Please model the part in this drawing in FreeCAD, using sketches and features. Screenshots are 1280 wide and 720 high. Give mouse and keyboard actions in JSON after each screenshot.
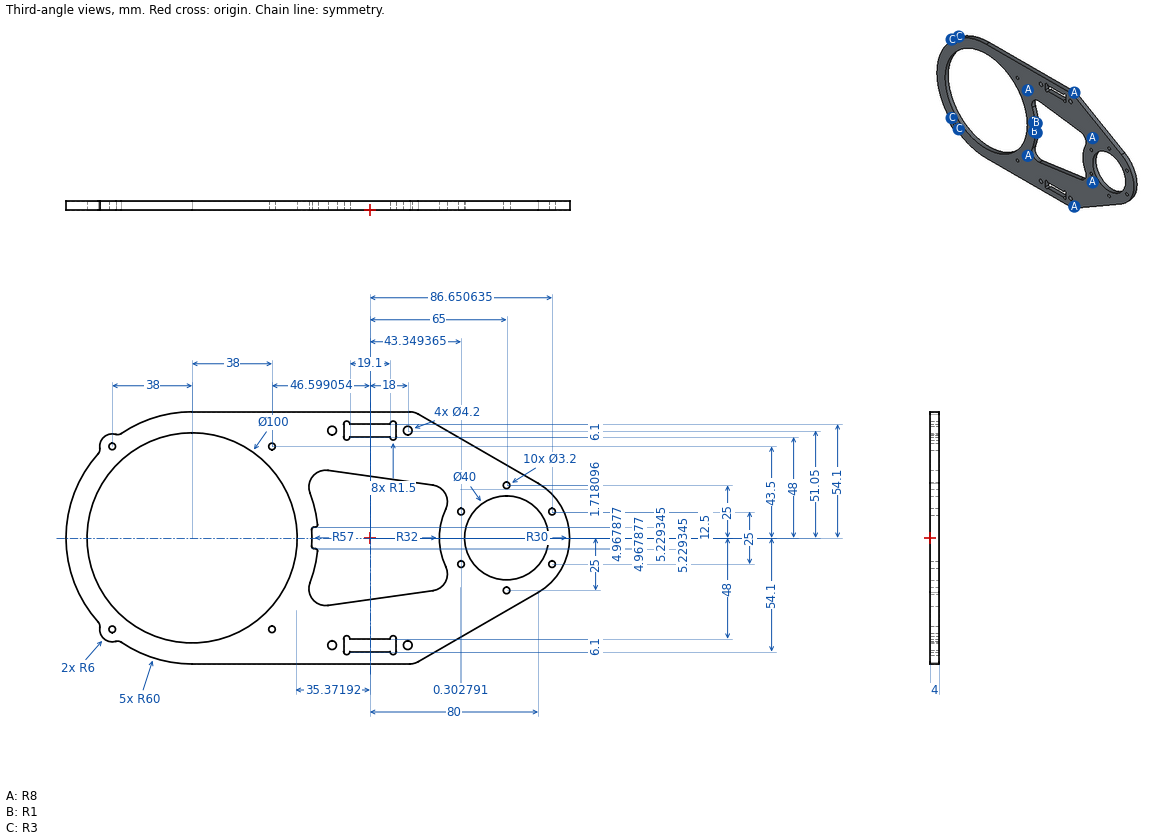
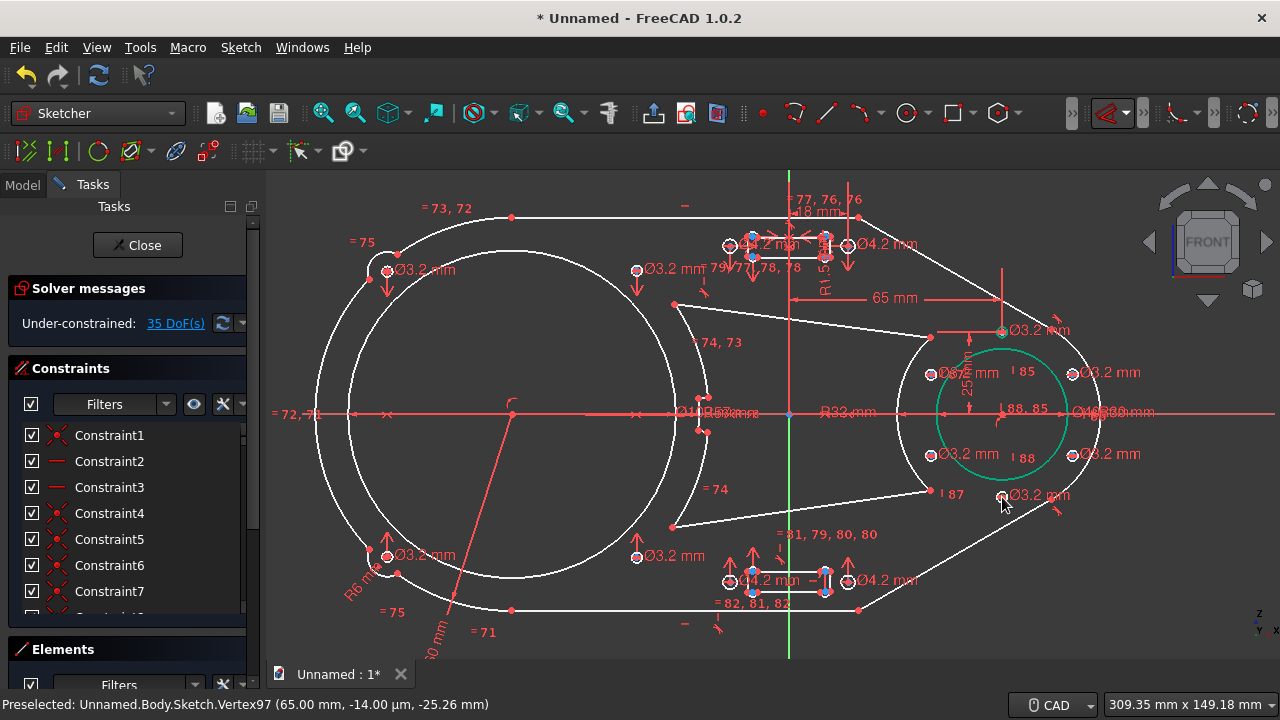
{"action": "left_click", "coordinate": [1128, 114]}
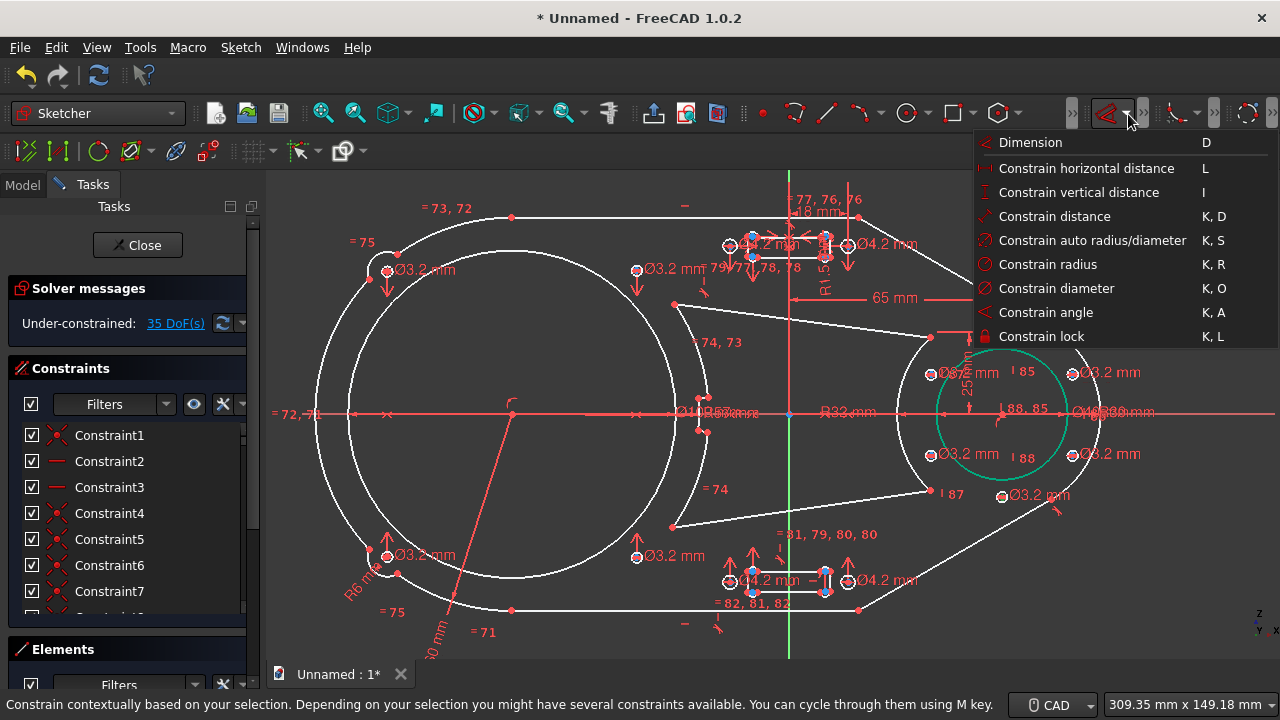
{"action": "left_click", "coordinate": [1126, 192]}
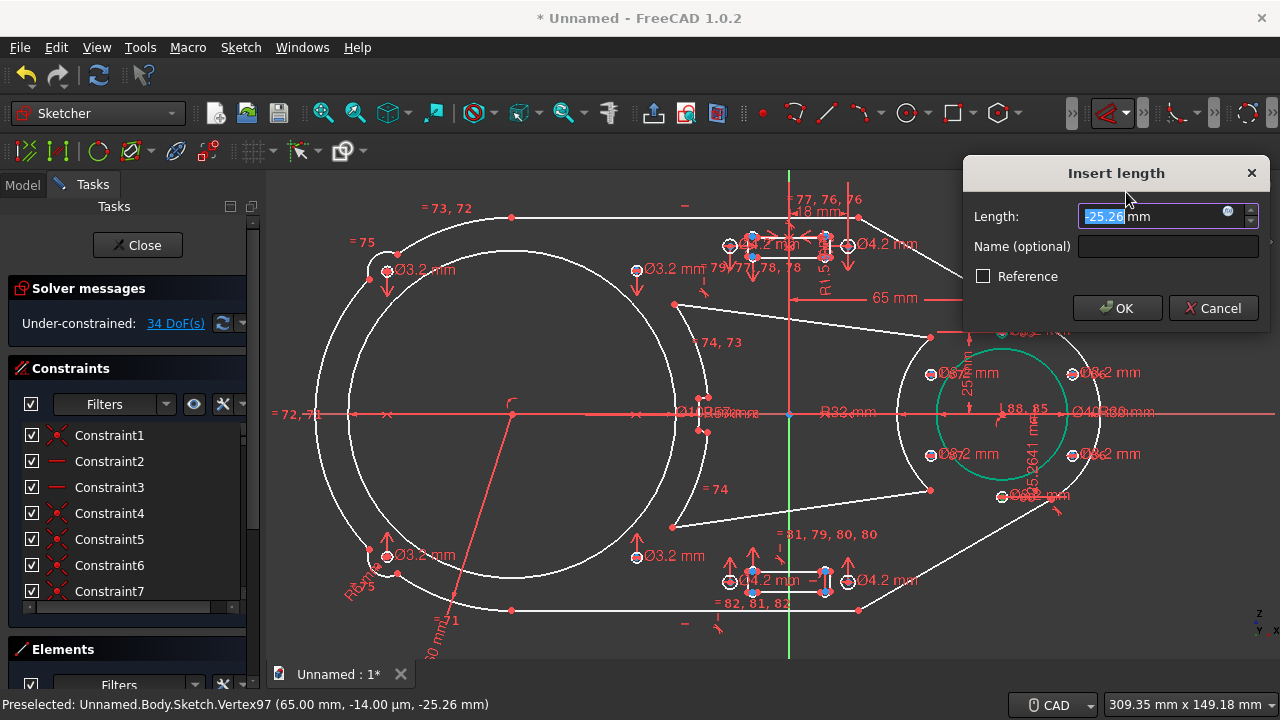
{"action": "type", "text": "-25"}
{"action": "key", "text": "Return"}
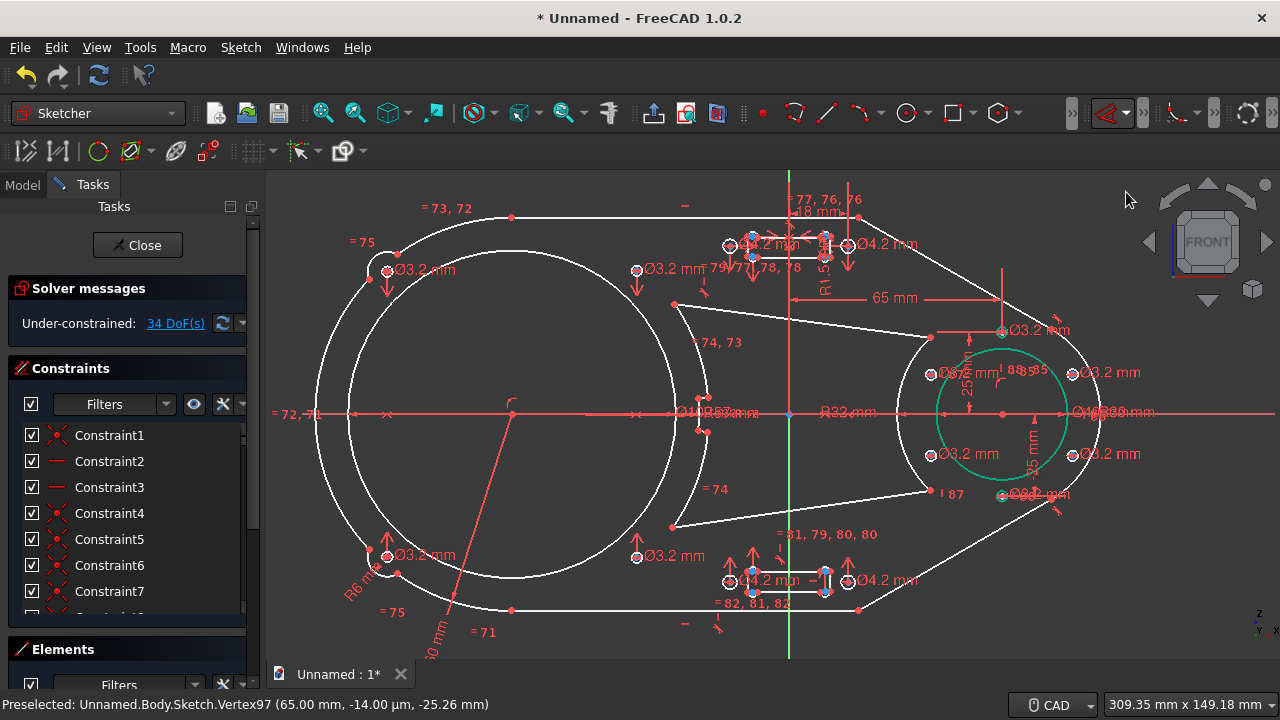
{"action": "scroll", "coordinate": [830, 247], "scroll_direction": "up", "scroll_amount": 4}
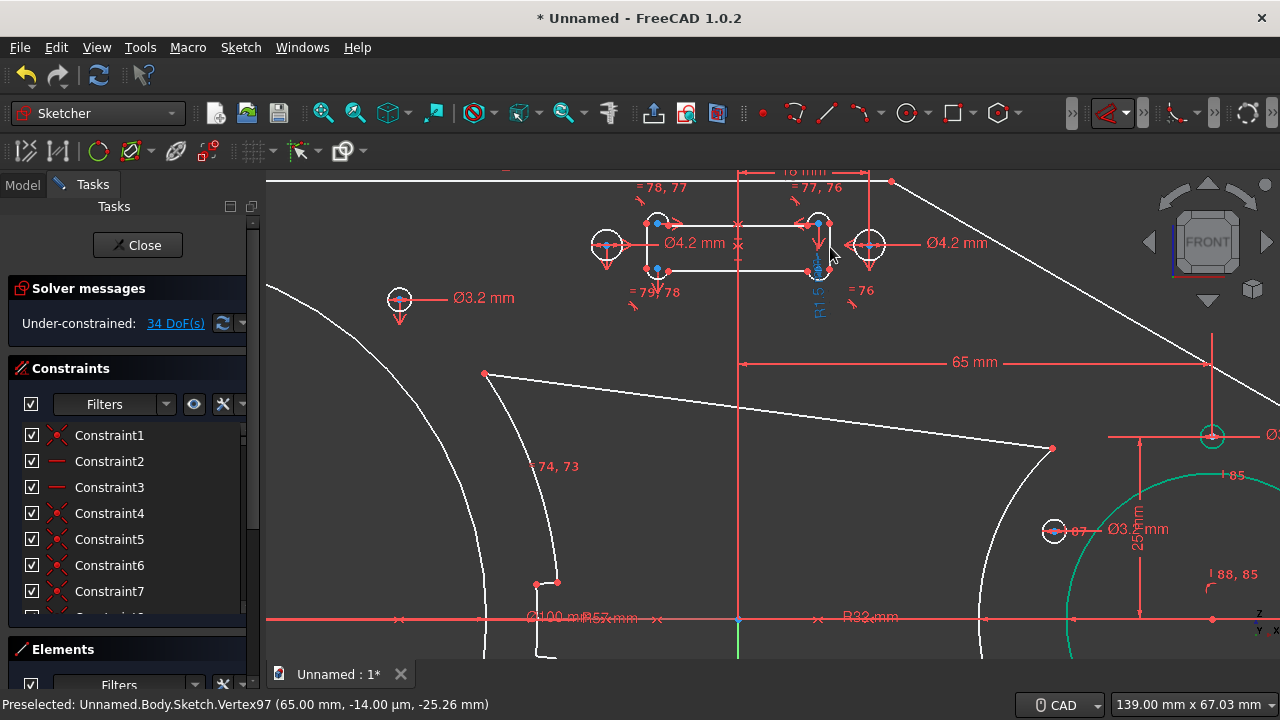
{"action": "left_click", "coordinate": [830, 247]}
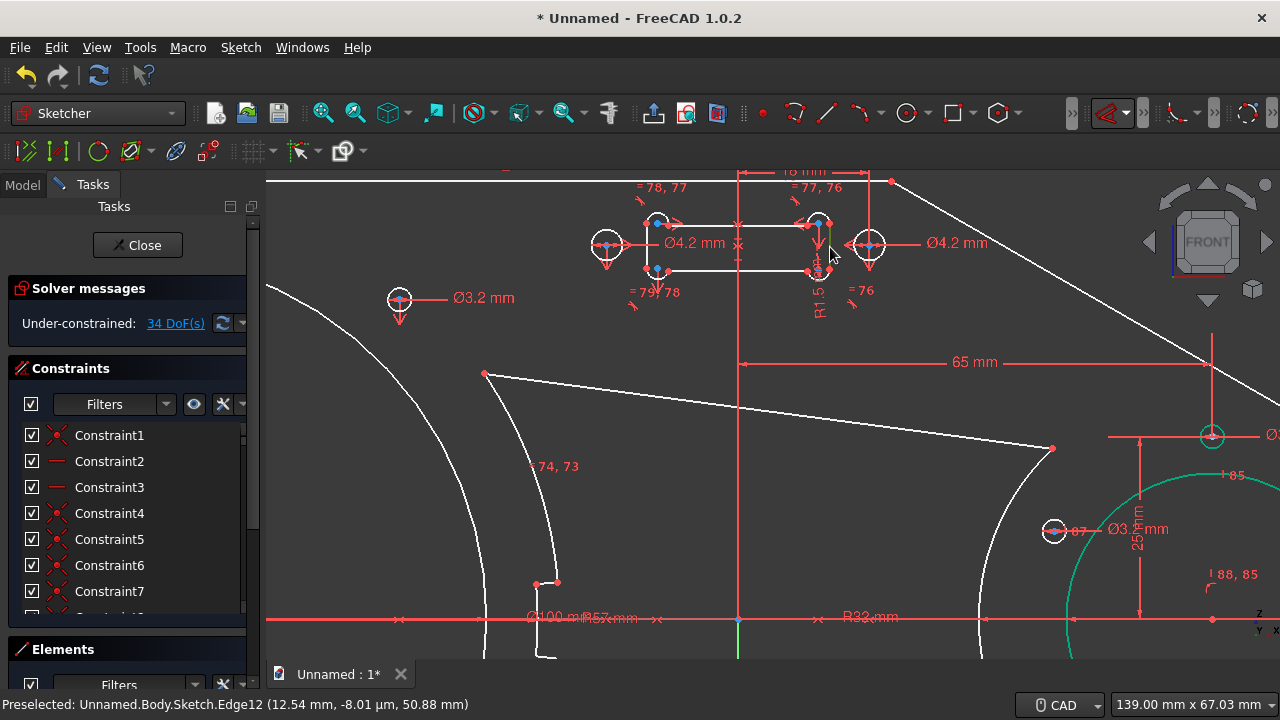
{"action": "key", "text": "i"}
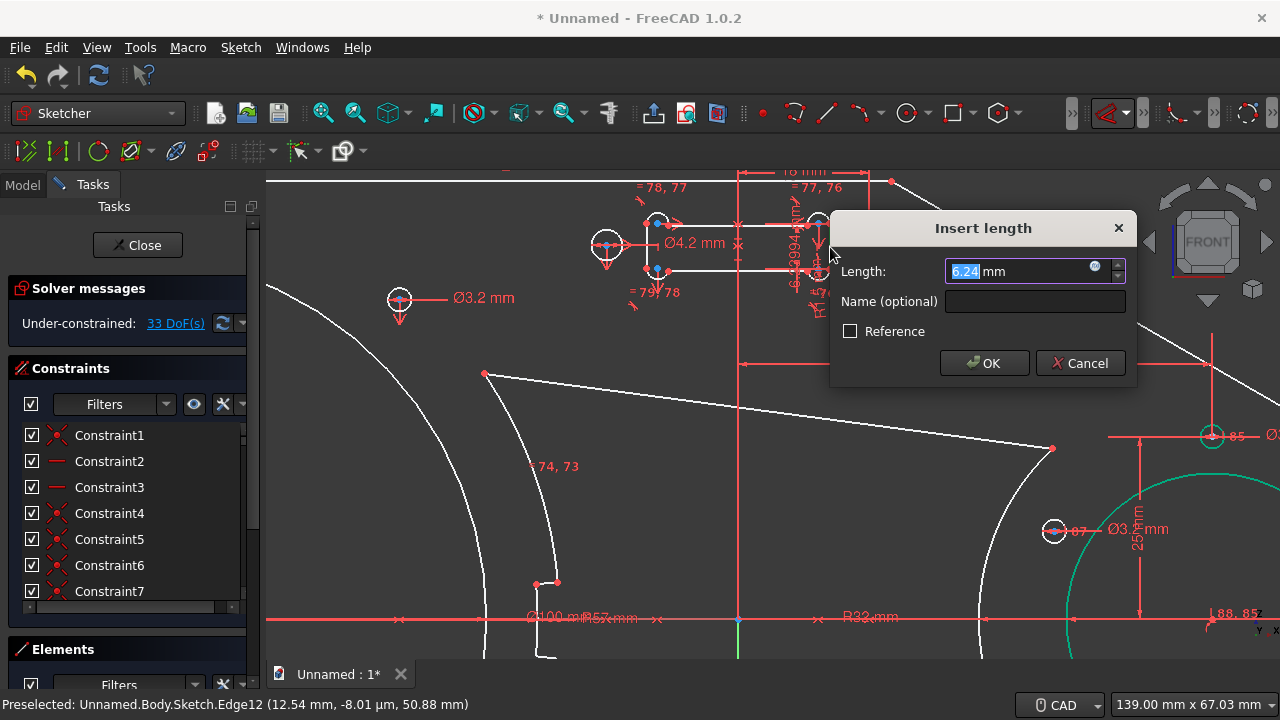
{"action": "type", "text": "6.1"}
{"action": "key", "text": "Return"}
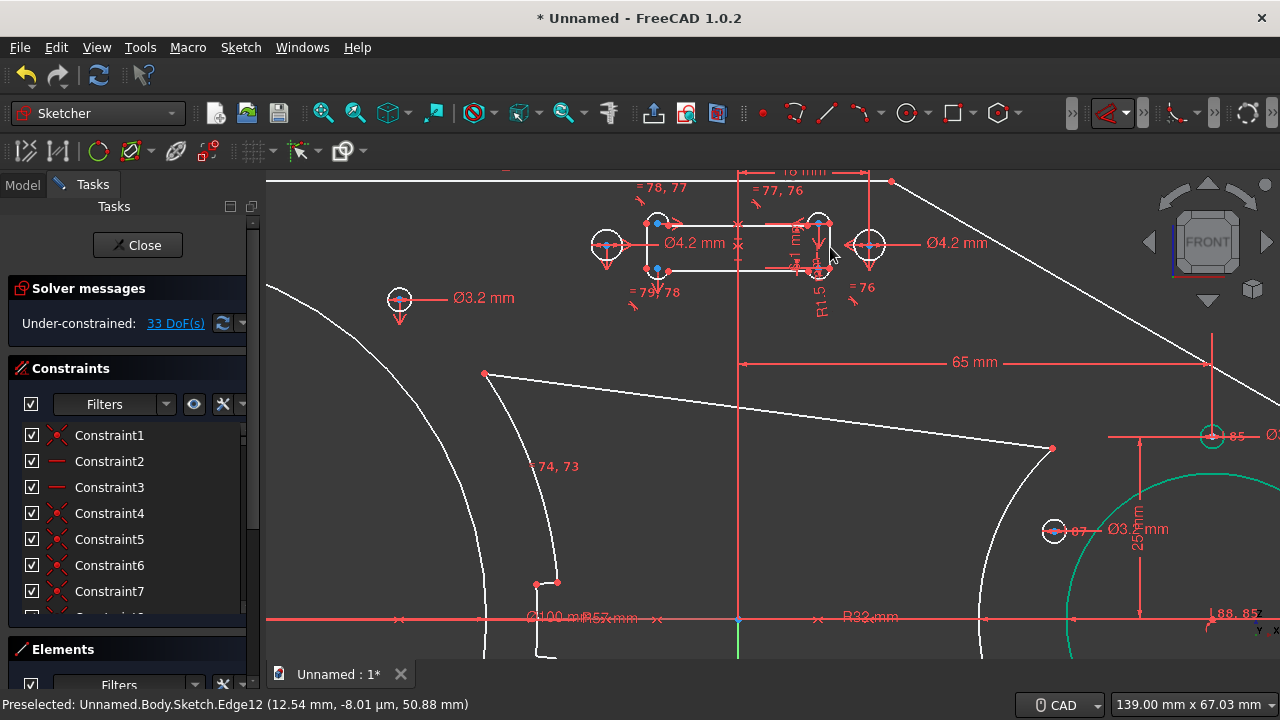
{"action": "left_click", "coordinate": [647, 237]}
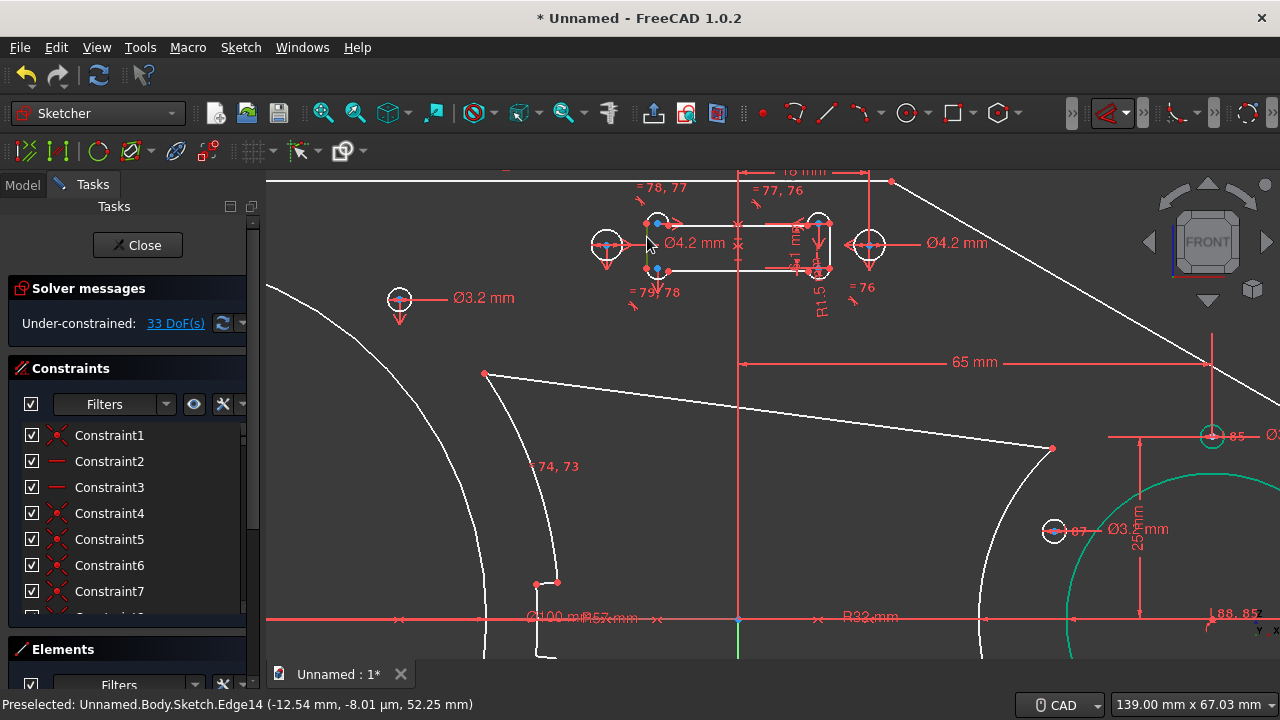
{"action": "left_click", "coordinate": [1128, 114]}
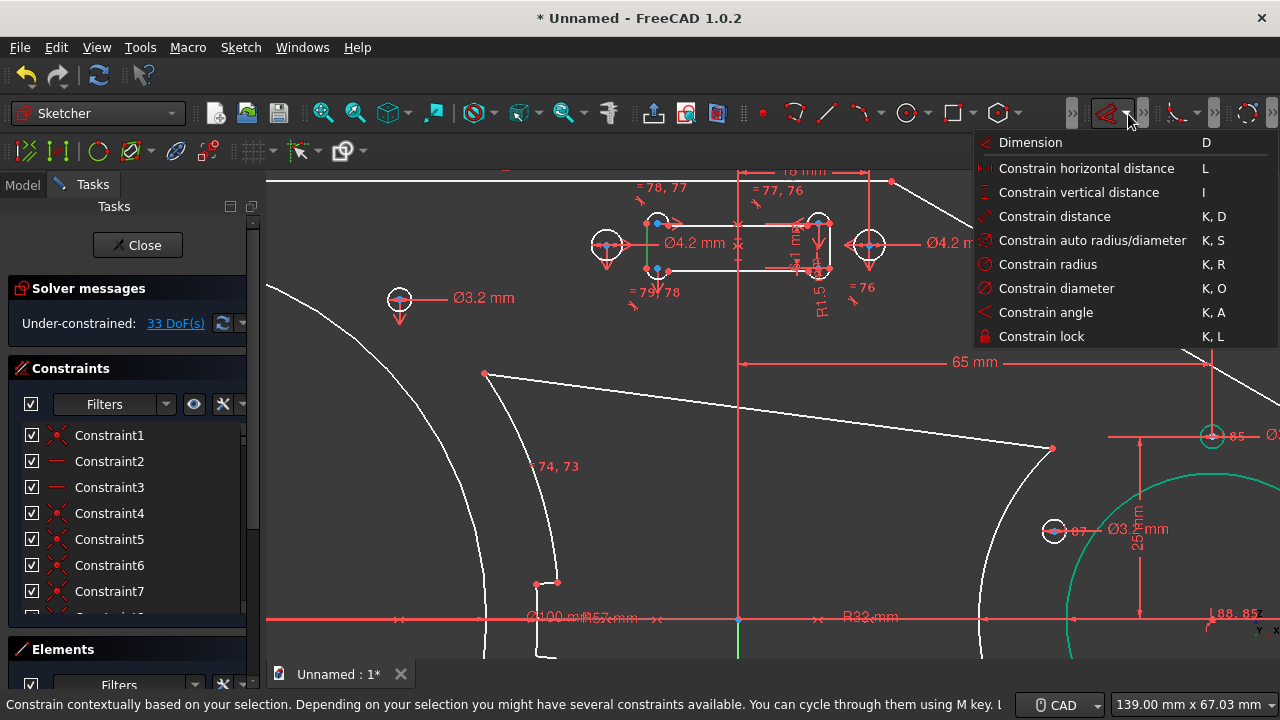
{"action": "left_click", "coordinate": [1126, 192]}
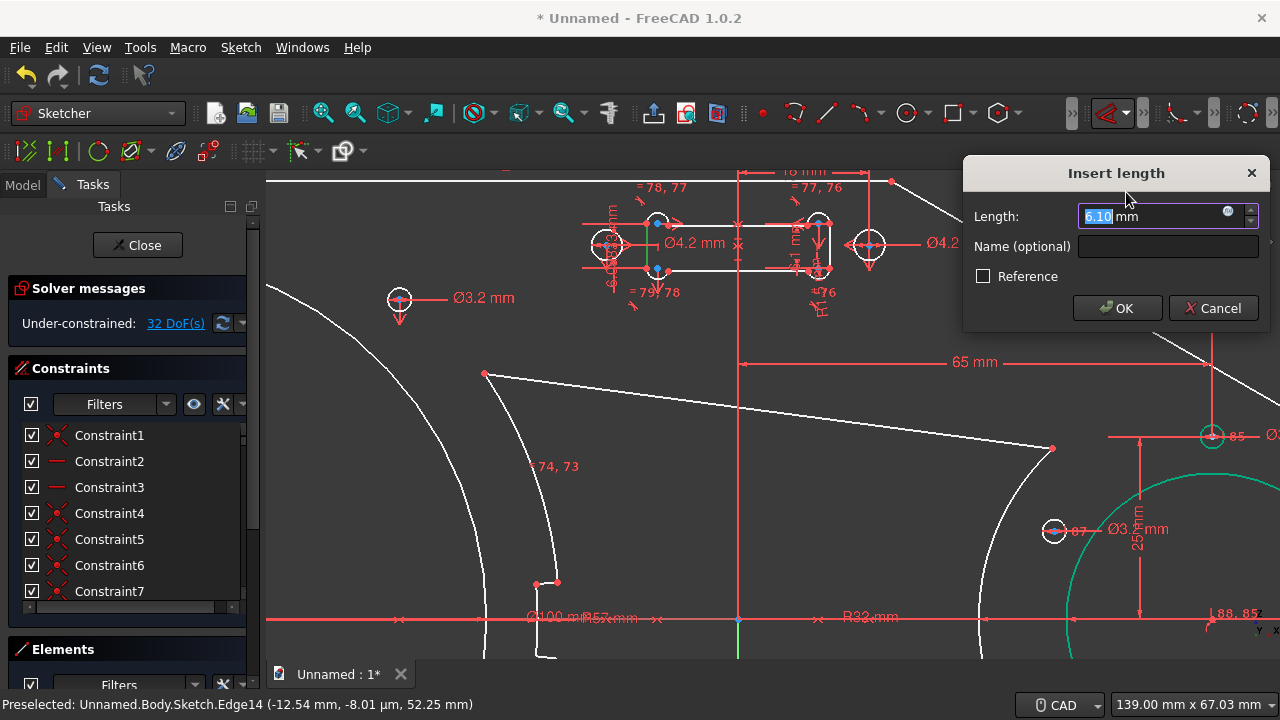
{"action": "type", "text": "6.1"}
{"action": "key", "text": "Return"}